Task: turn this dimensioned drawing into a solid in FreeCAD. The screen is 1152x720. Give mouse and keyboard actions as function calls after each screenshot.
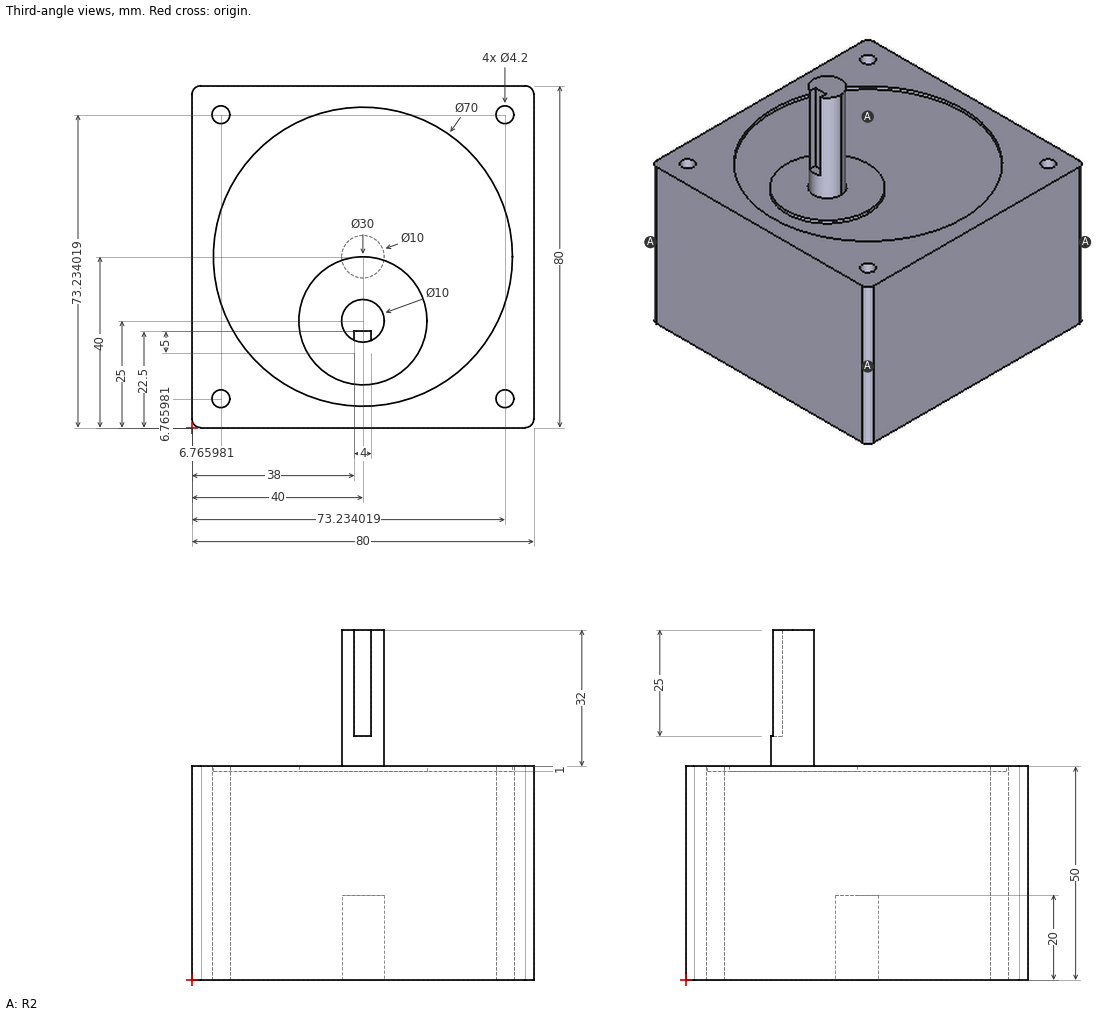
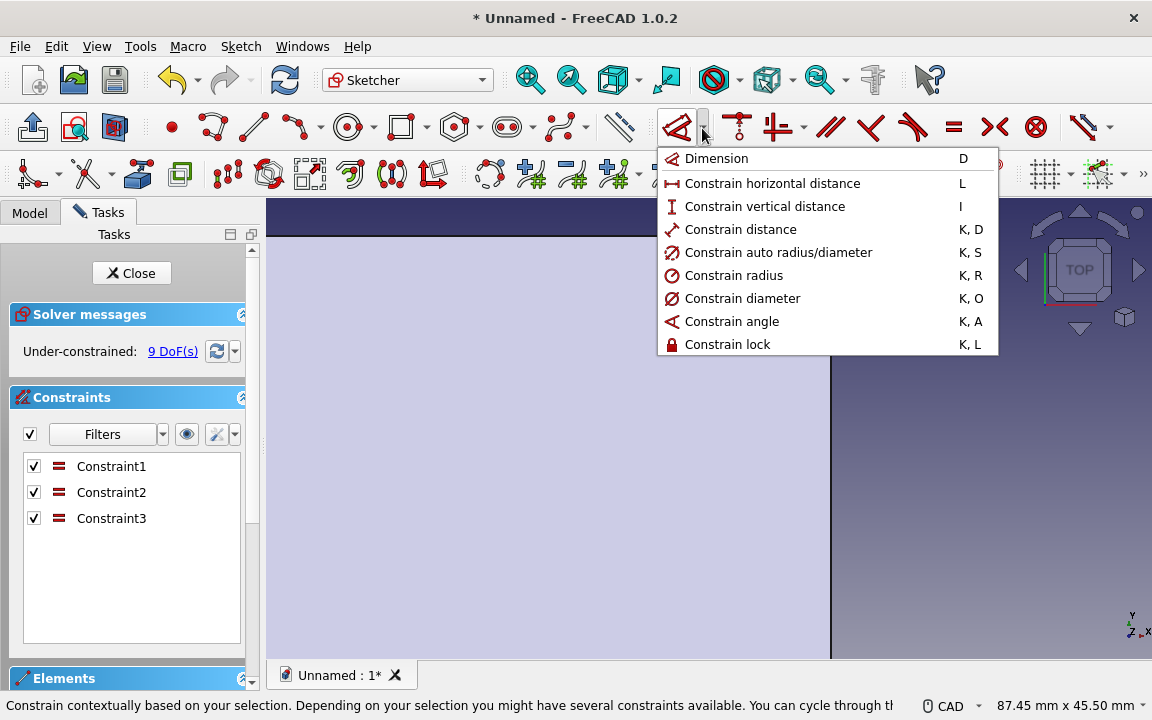
click(828, 298)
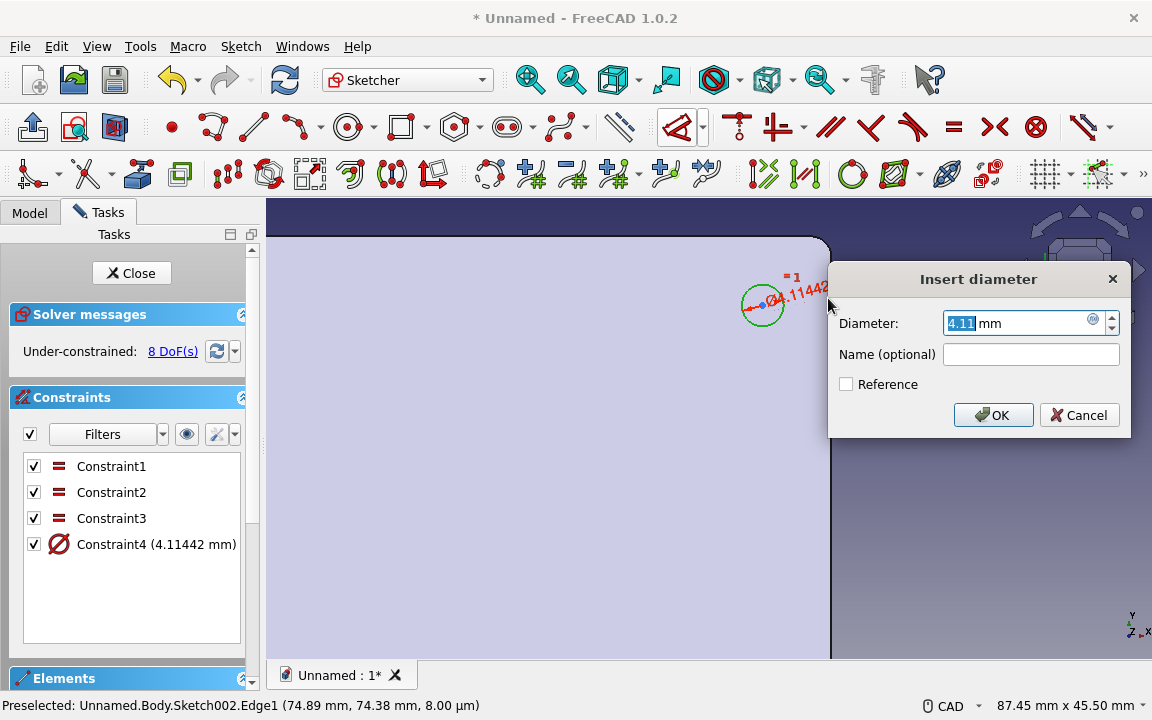
text(4.2)
key(Return)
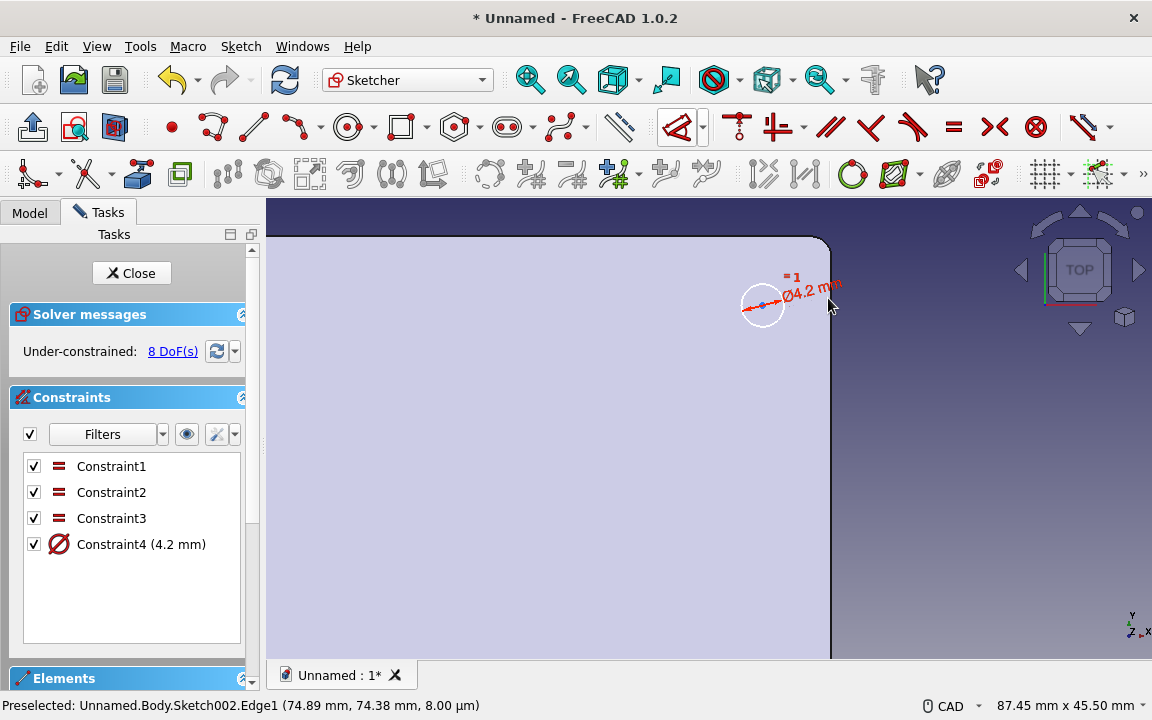
scroll(779, 291, down, 5)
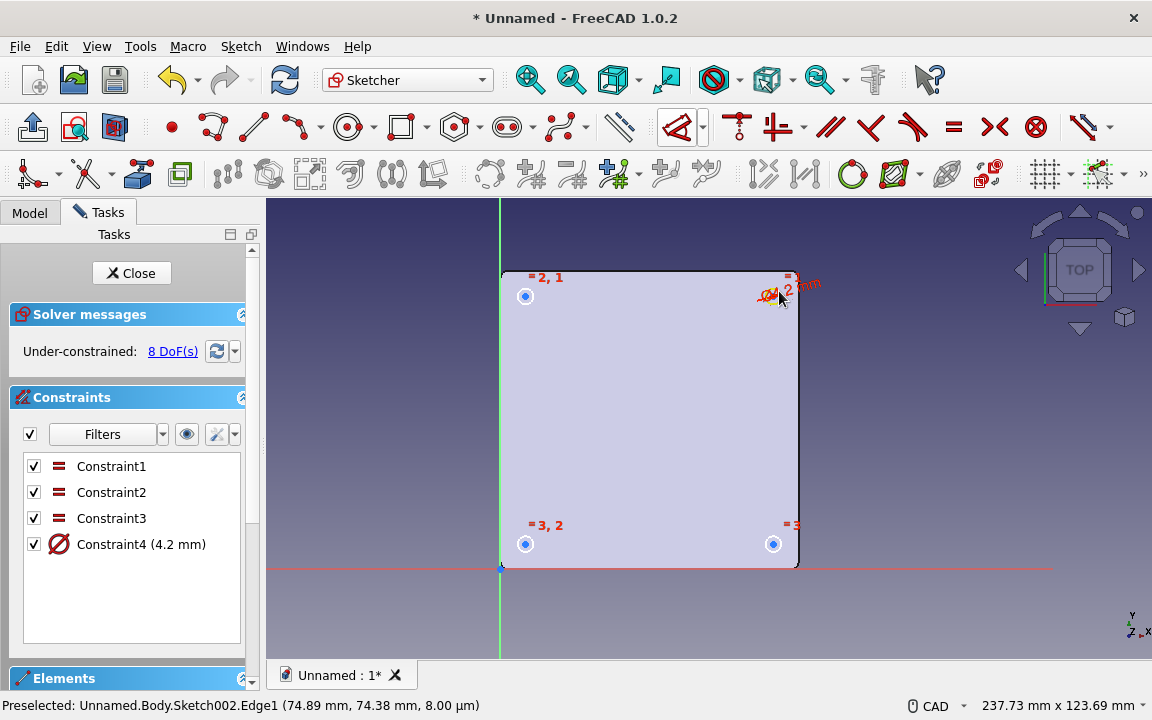
scroll(526, 296, up, 3)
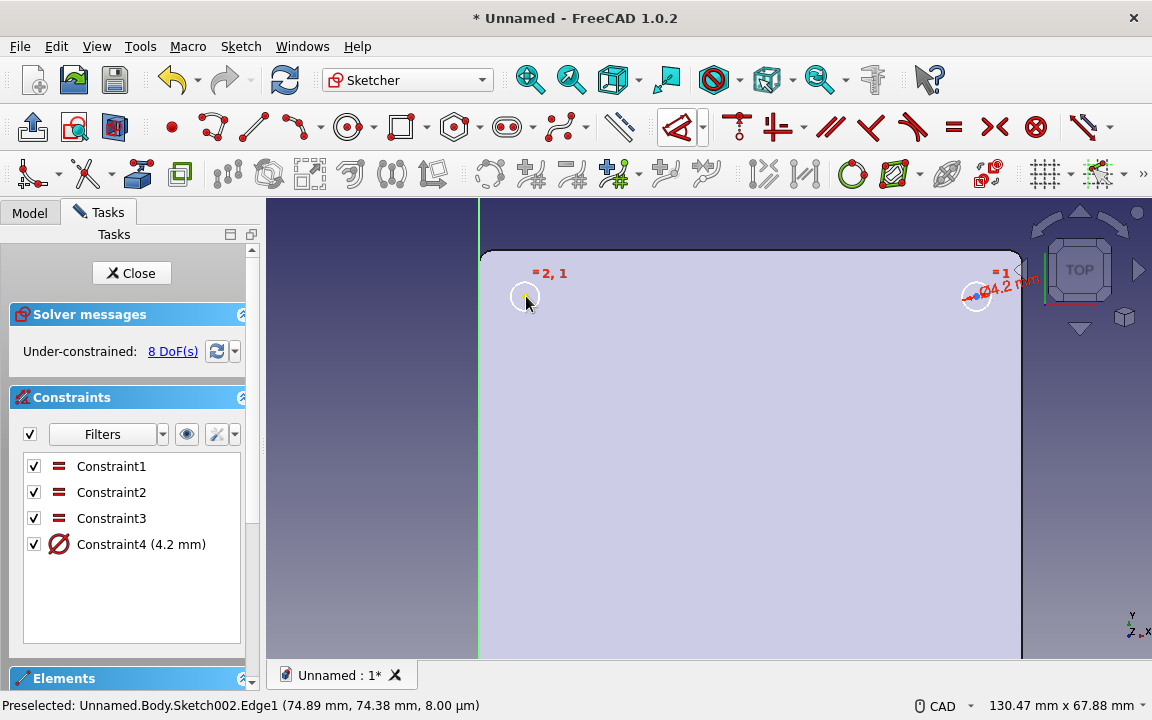
click(525, 297)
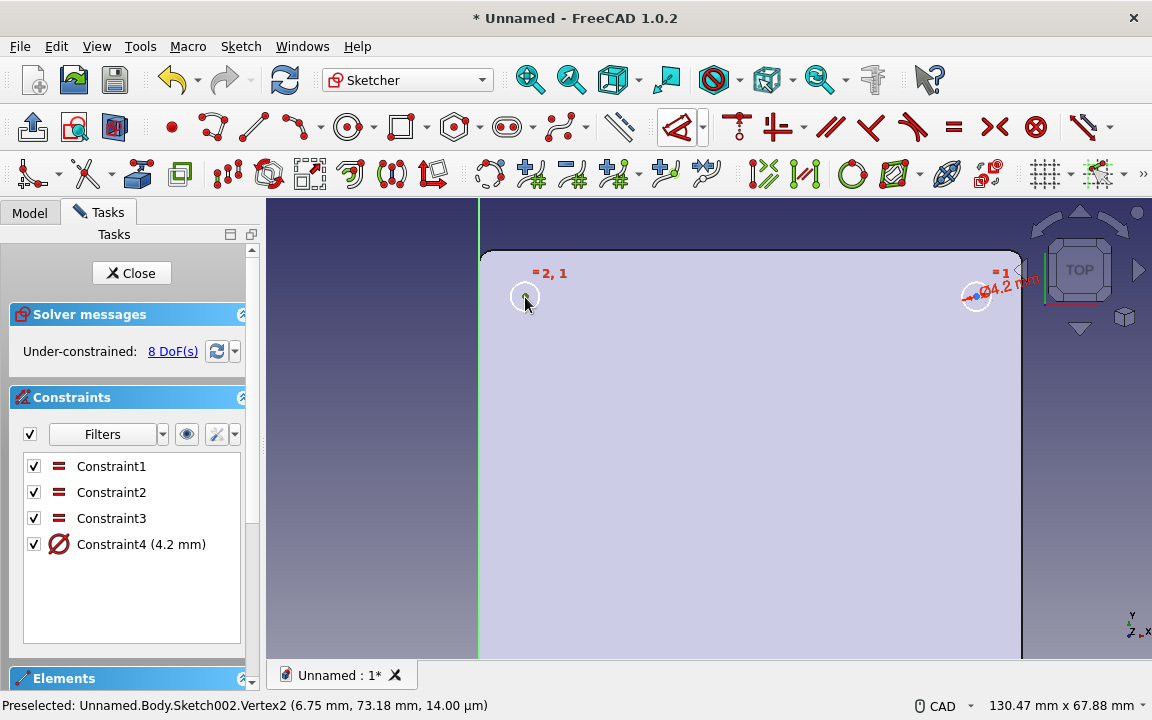
click(702, 128)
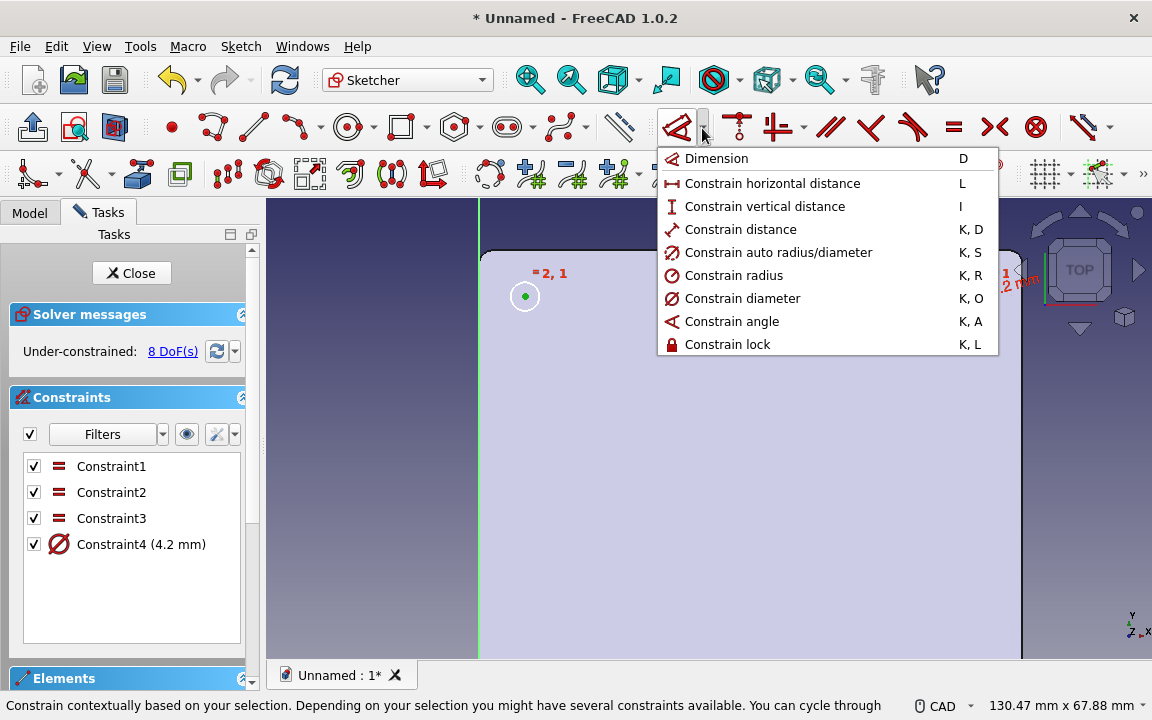
click(828, 184)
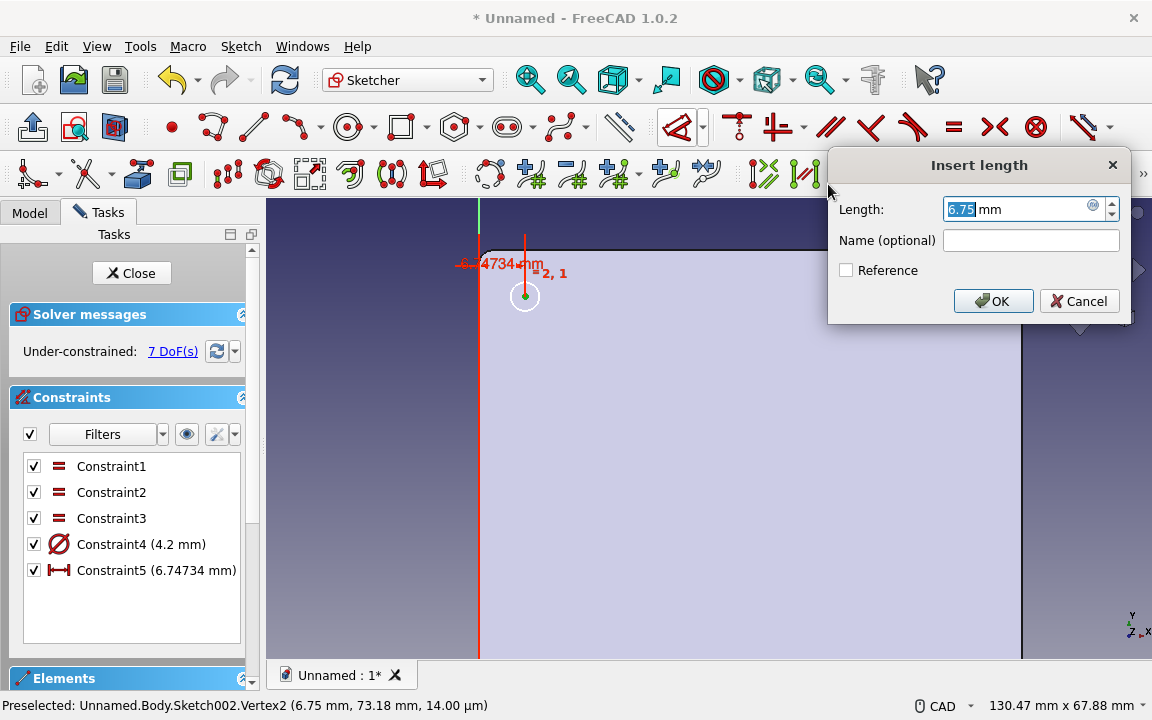
text(6.765981)
key(Return)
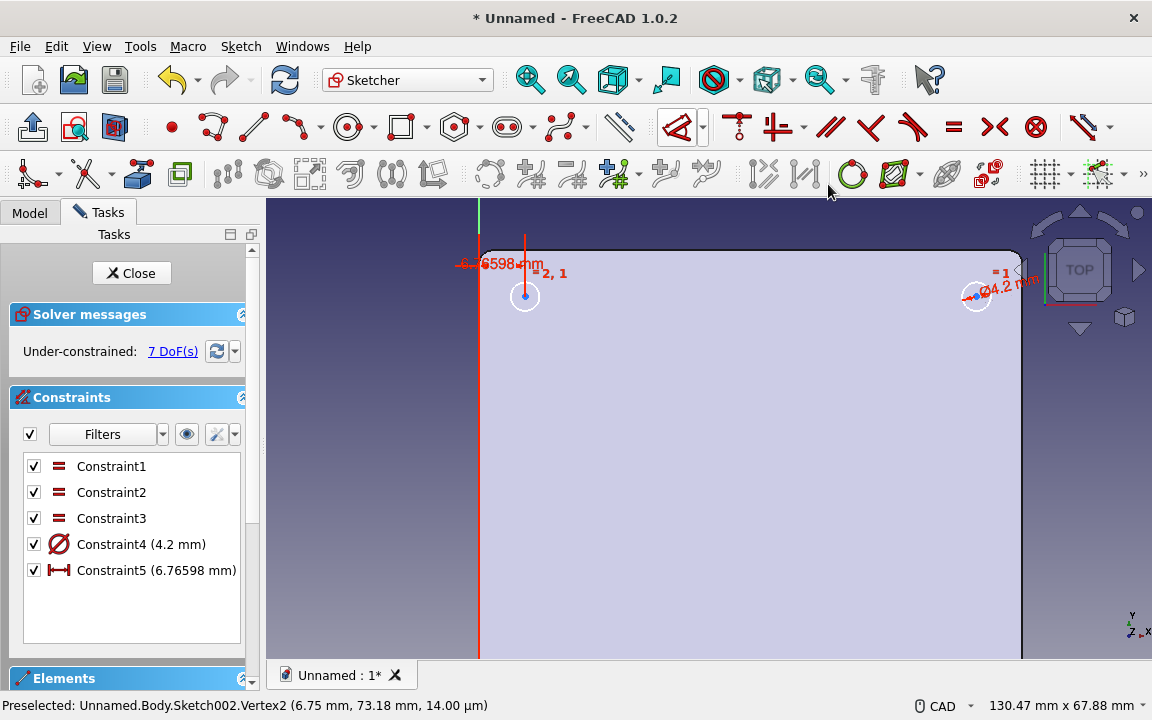
scroll(526, 296, down, 3)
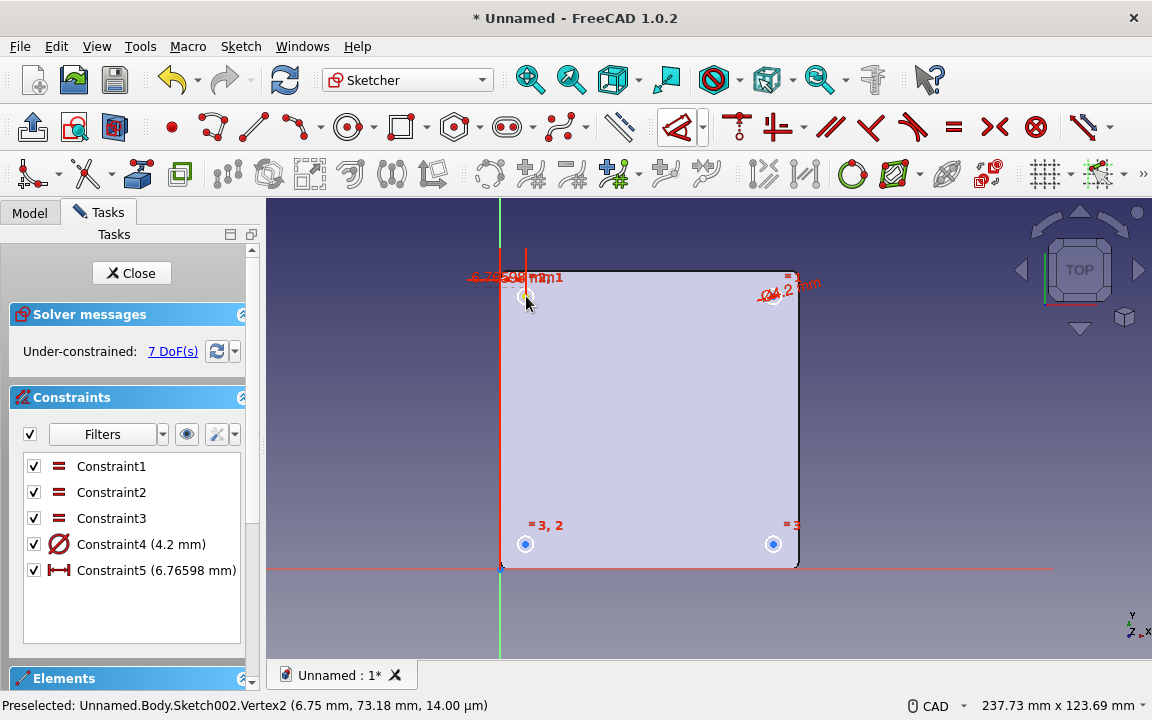
scroll(526, 544, up, 3)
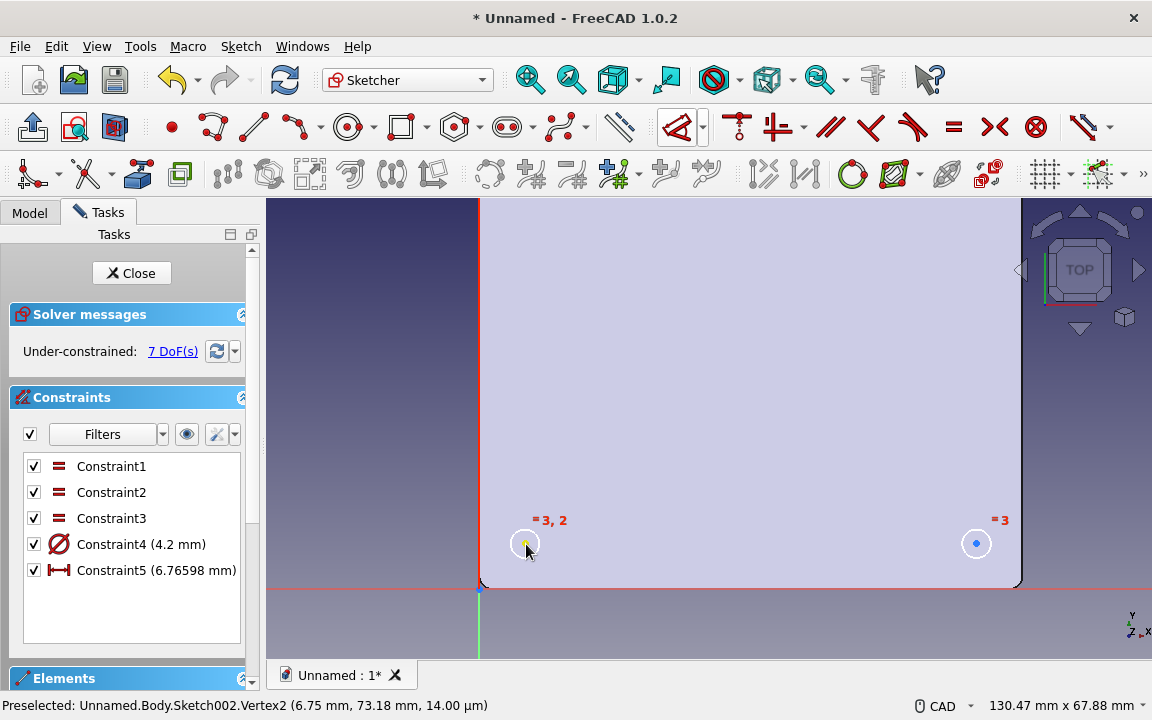
click(525, 544)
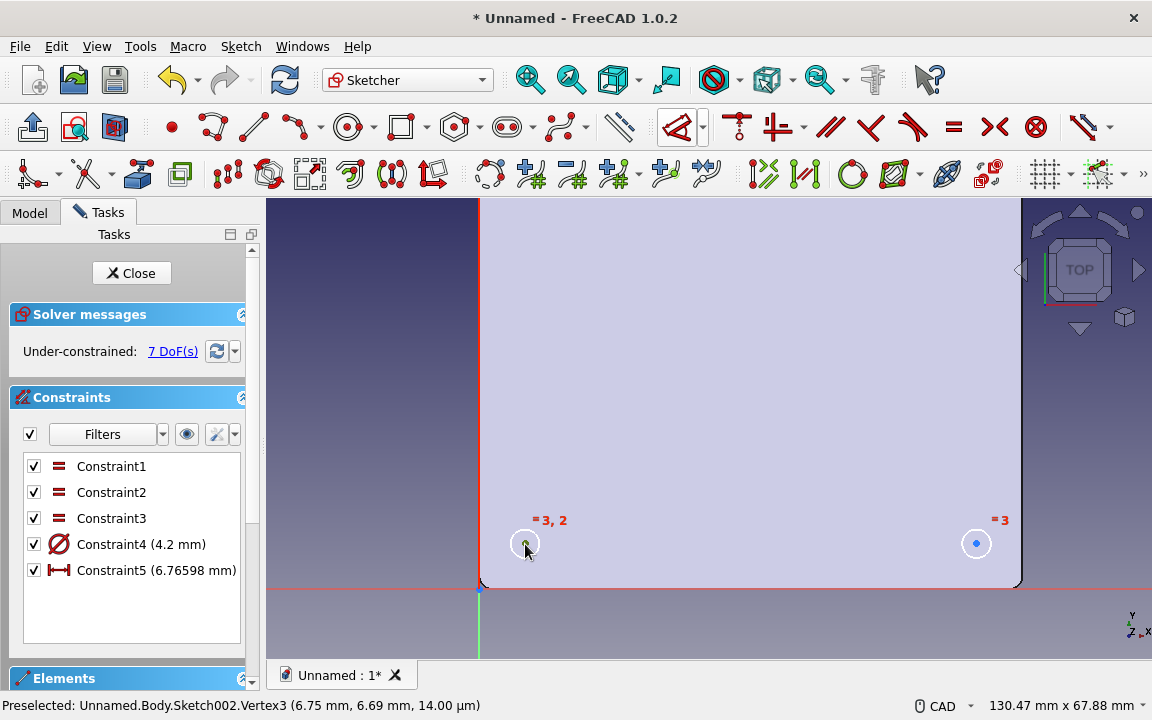
click(702, 128)